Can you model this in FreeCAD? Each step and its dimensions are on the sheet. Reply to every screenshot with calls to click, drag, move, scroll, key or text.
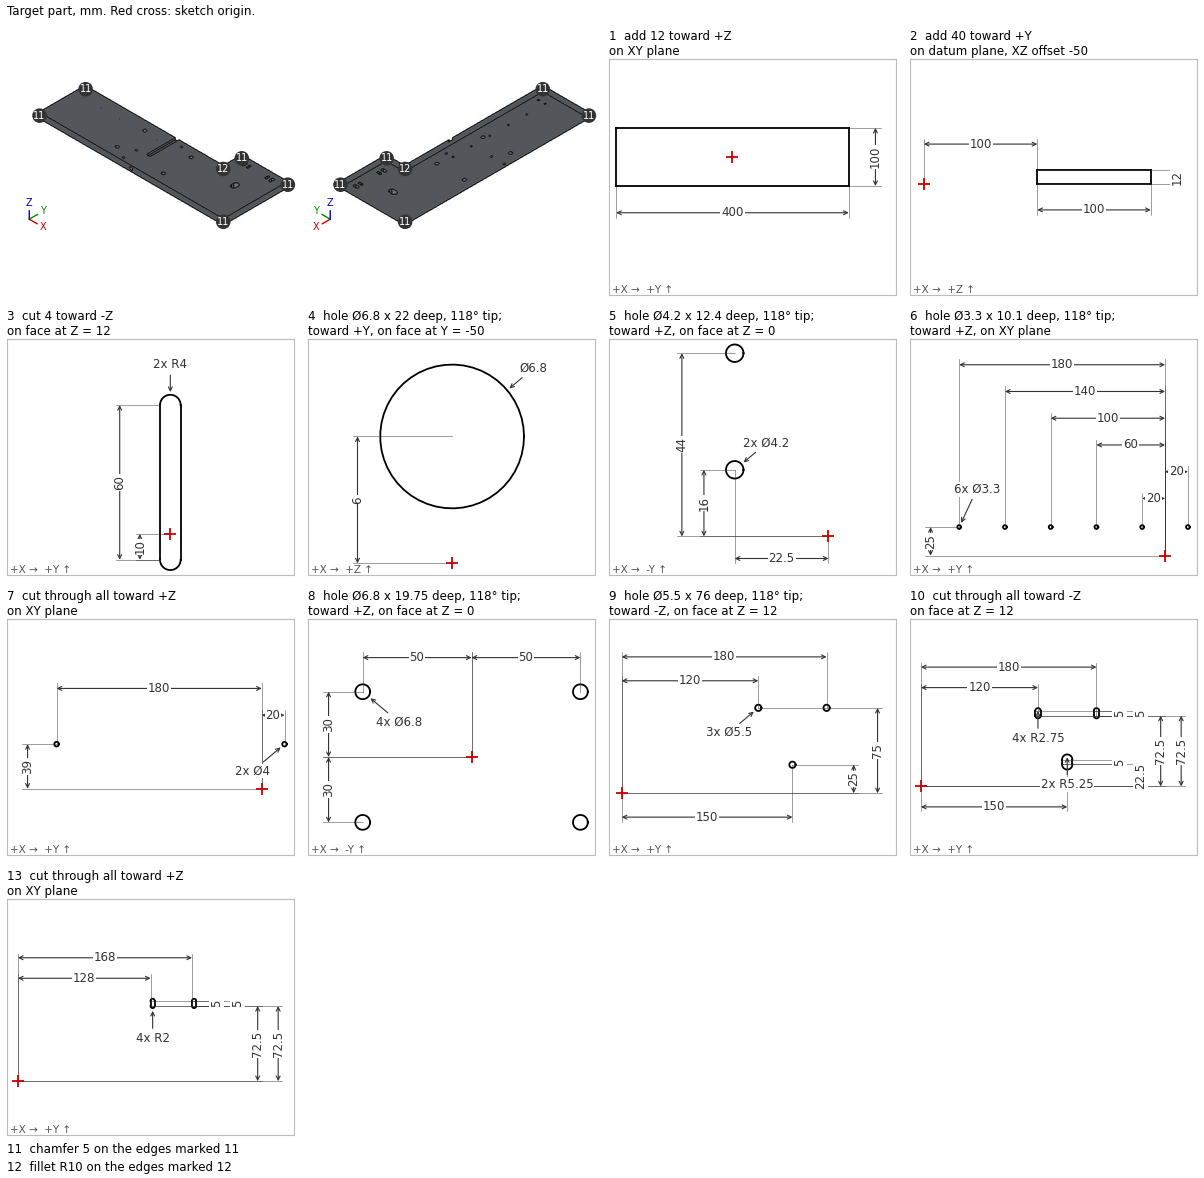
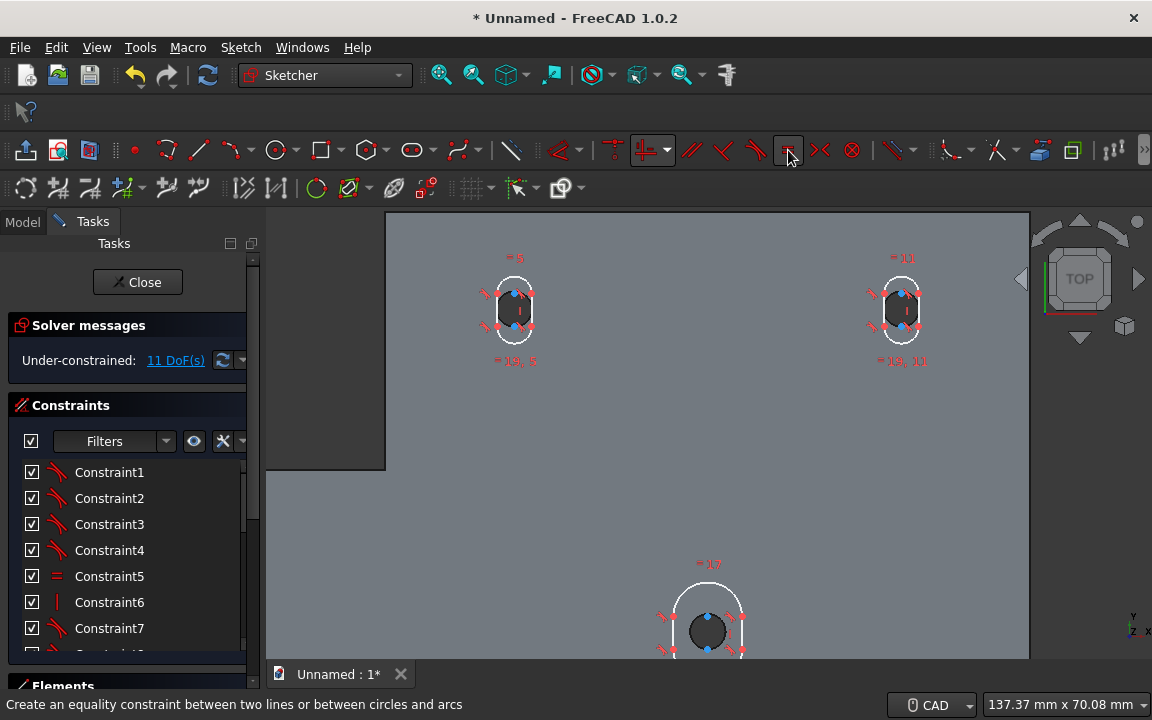
click(558, 150)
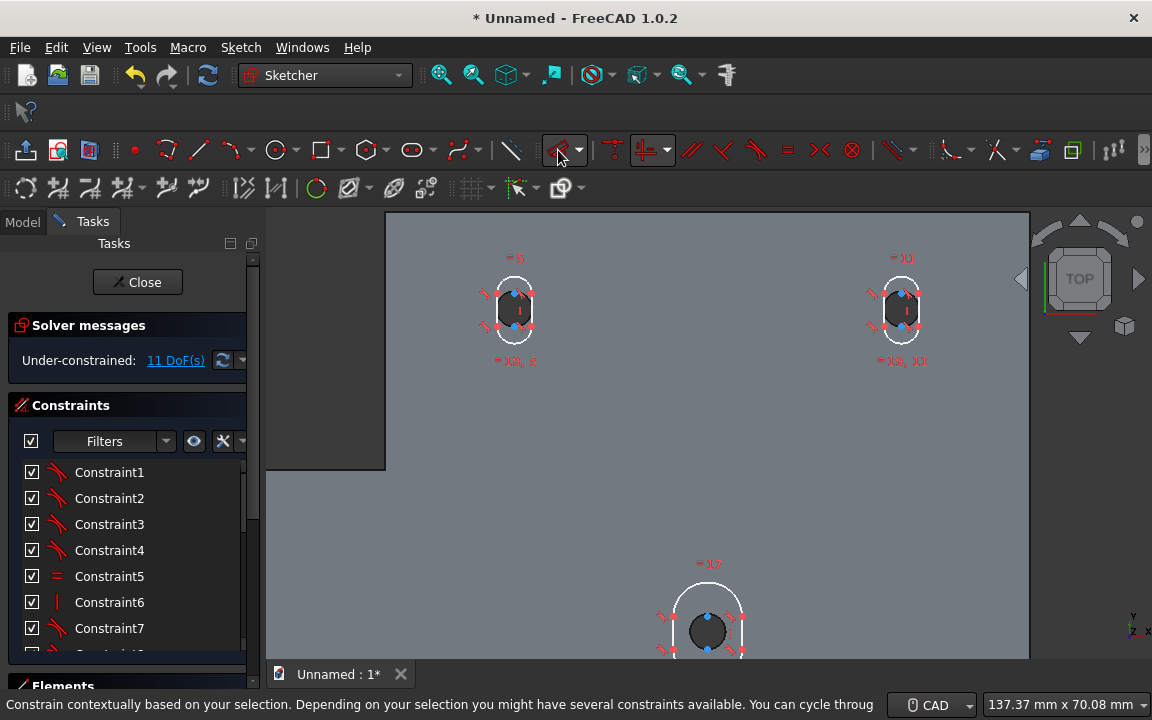
scroll(504, 340, up, 5)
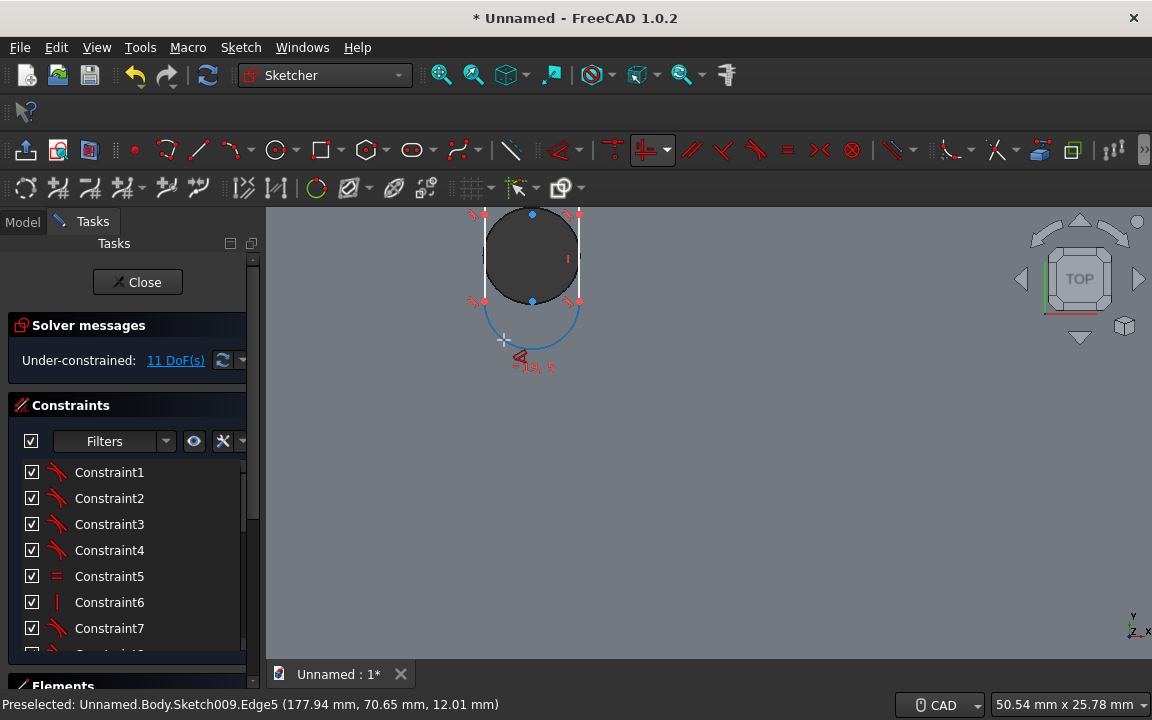
click(504, 340)
click(485, 366)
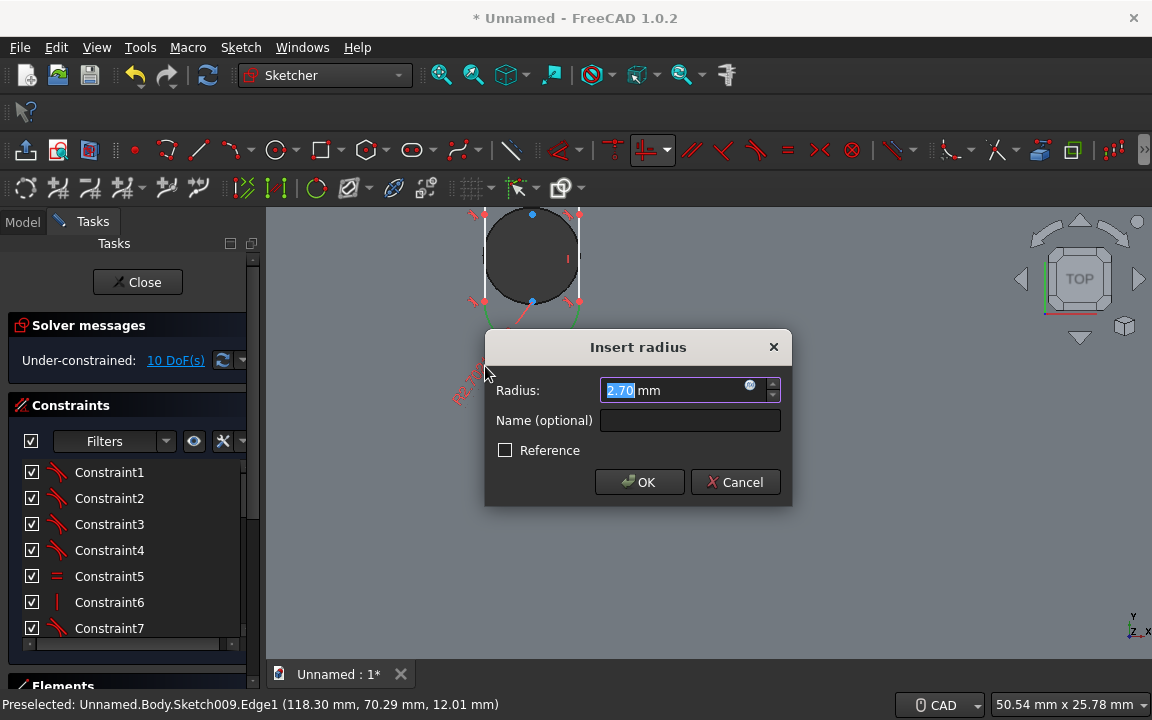
text(2.75)
key(Return)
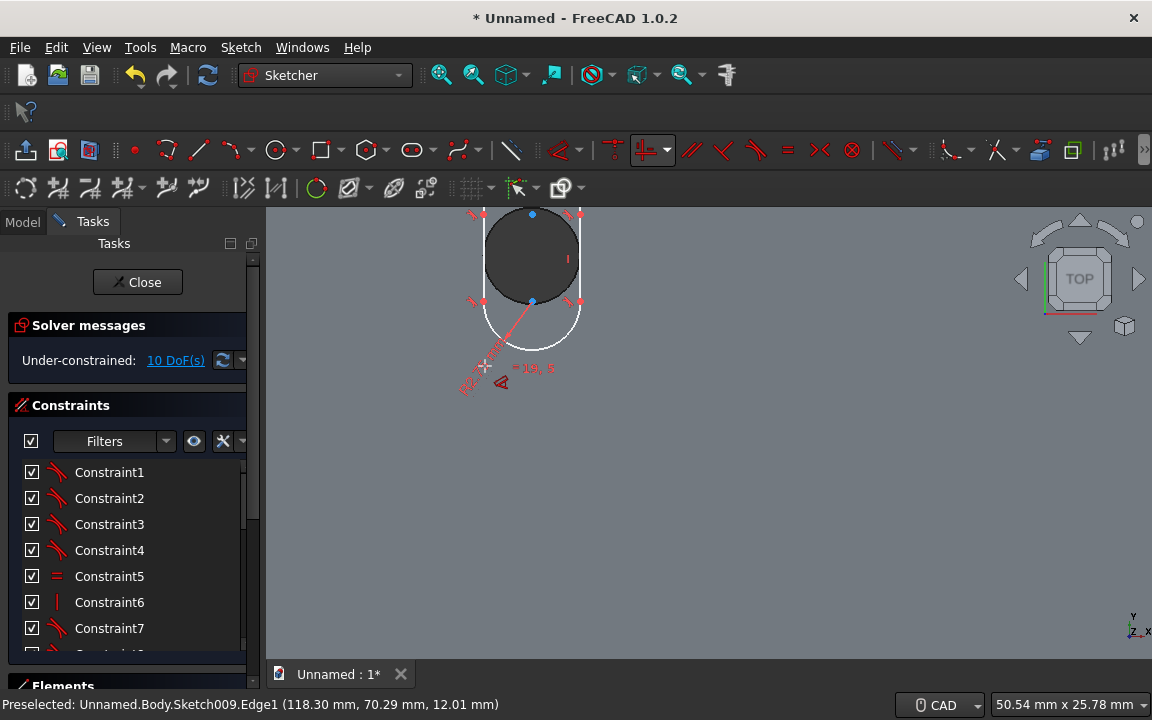
scroll(504, 340, down, 7)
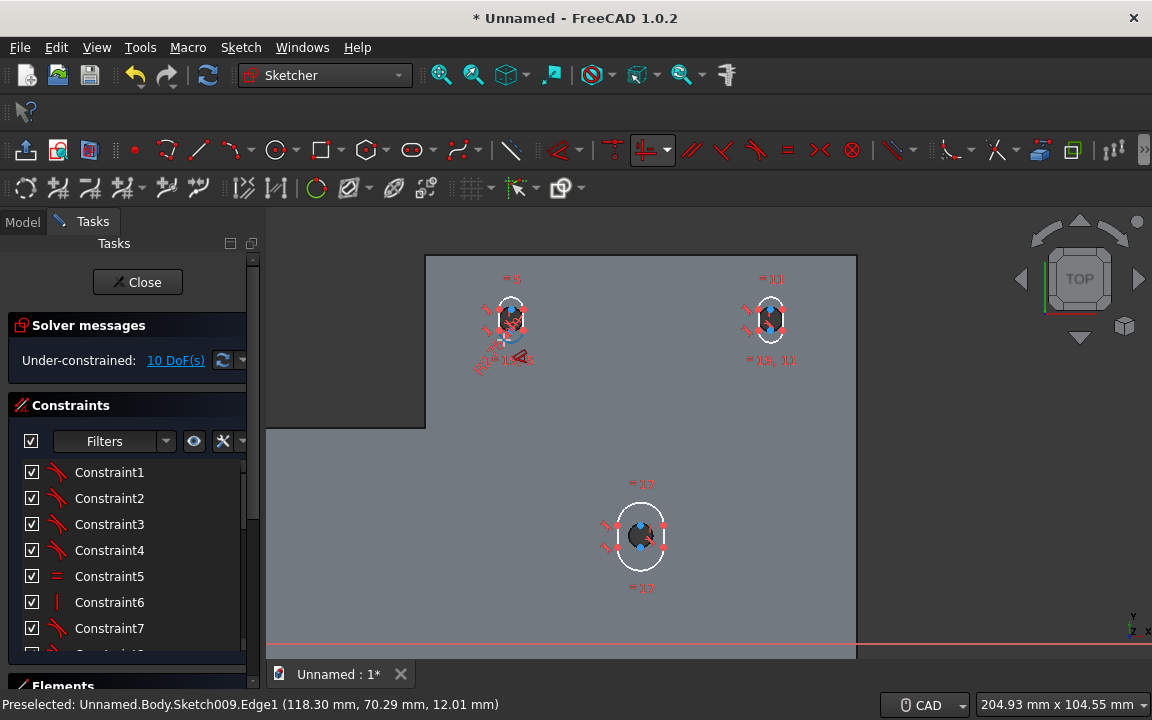
scroll(627, 566, up, 3)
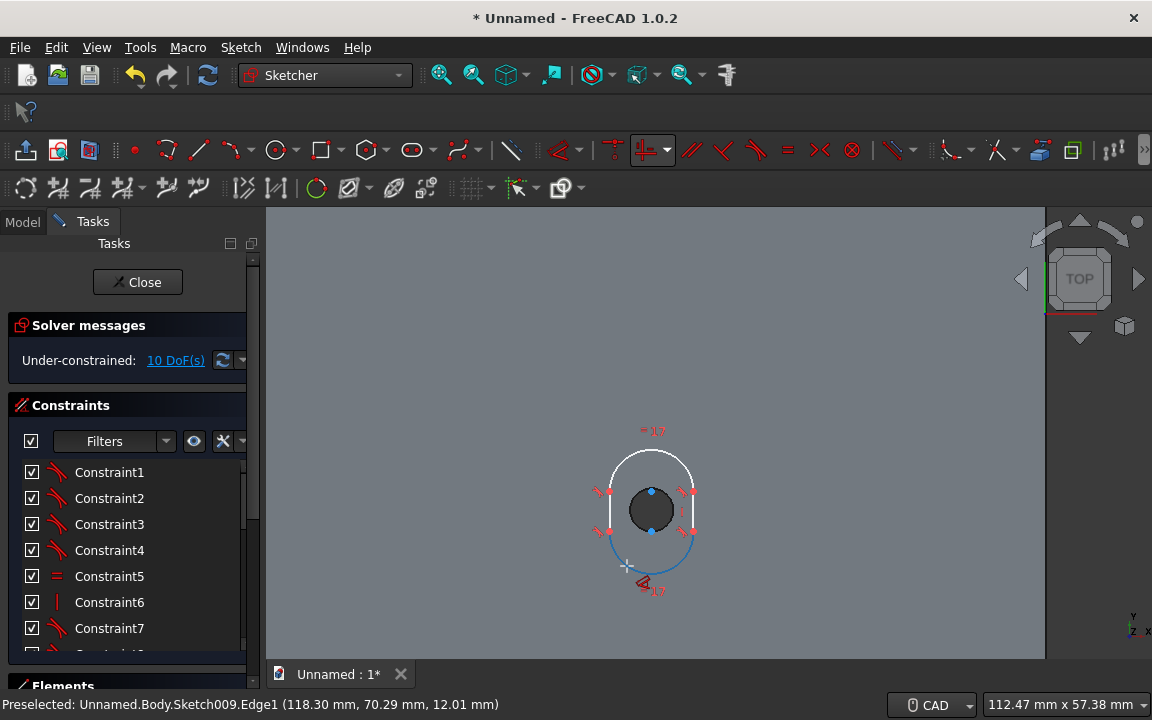
click(627, 566)
click(608, 592)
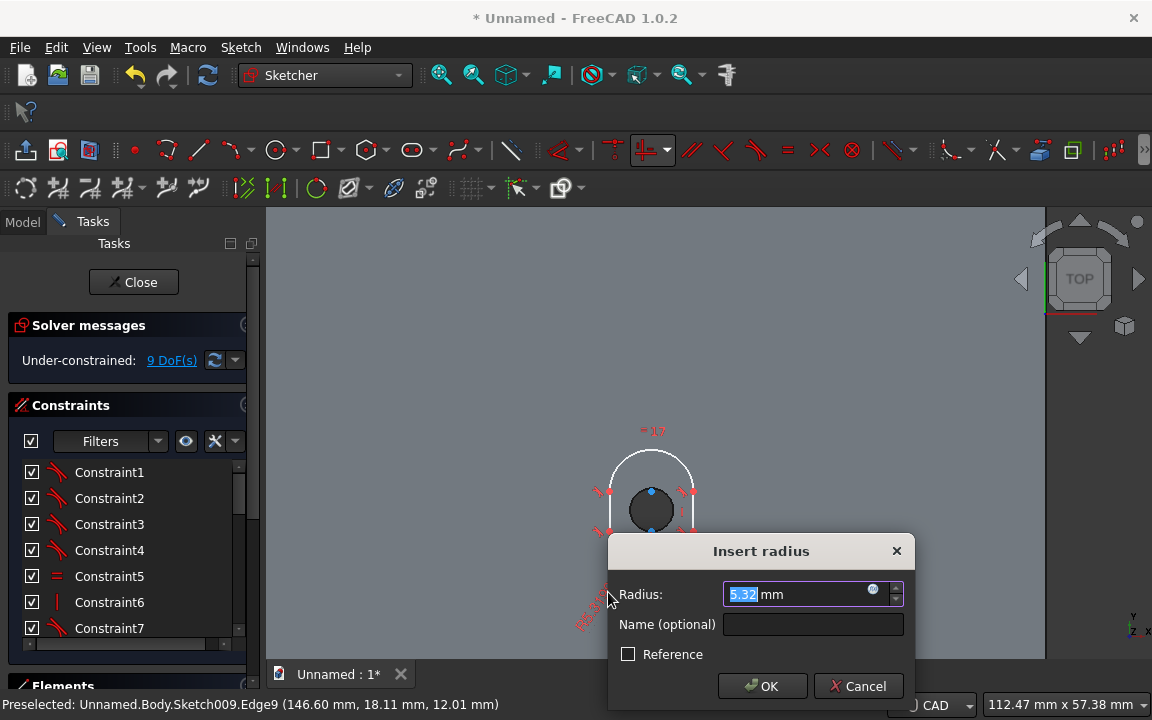
text(5.25)
key(Return)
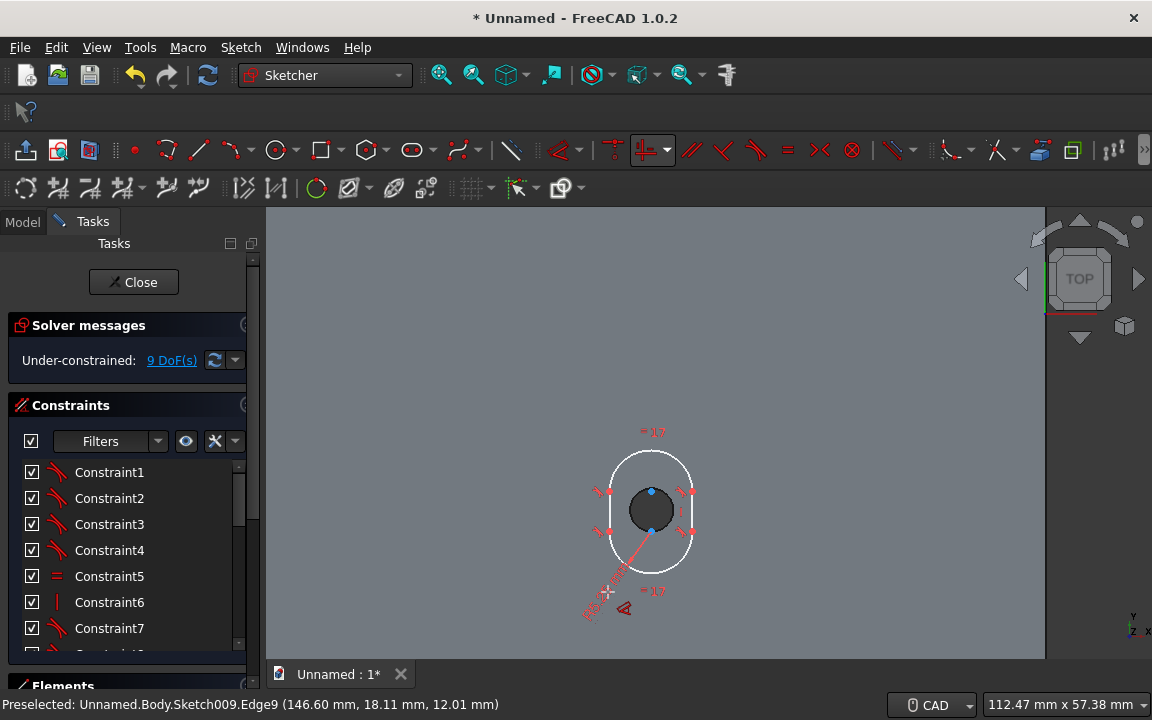
scroll(627, 567, down, 3)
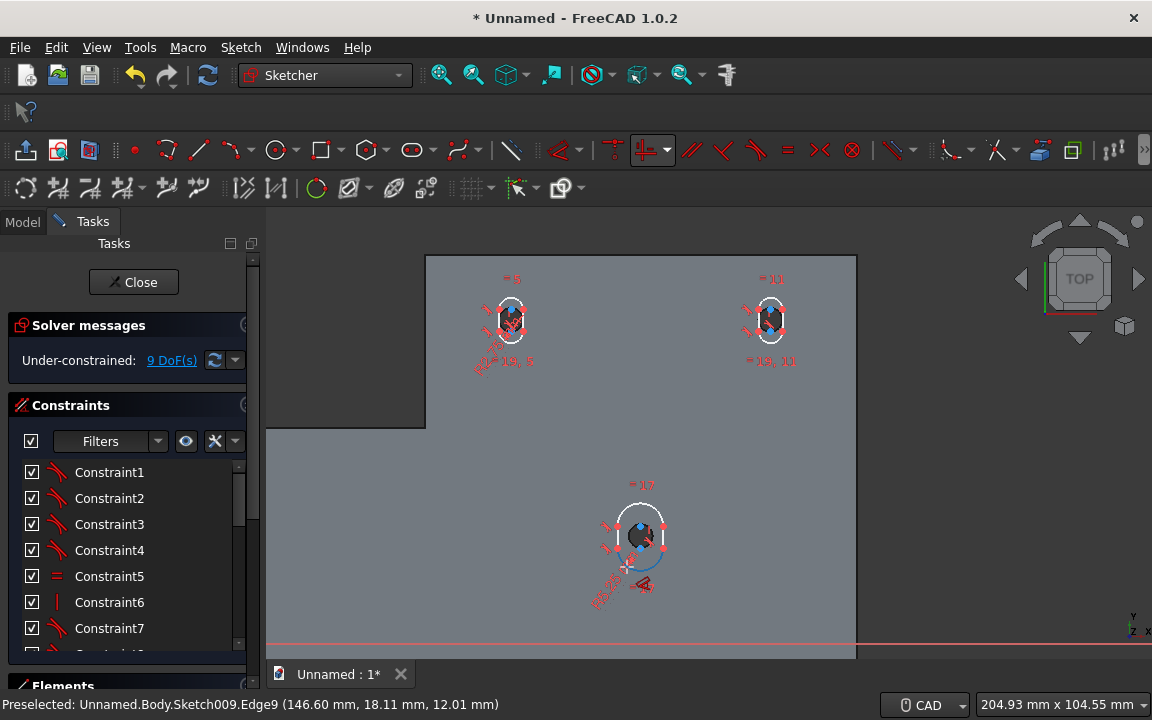
scroll(499, 325, up, 4)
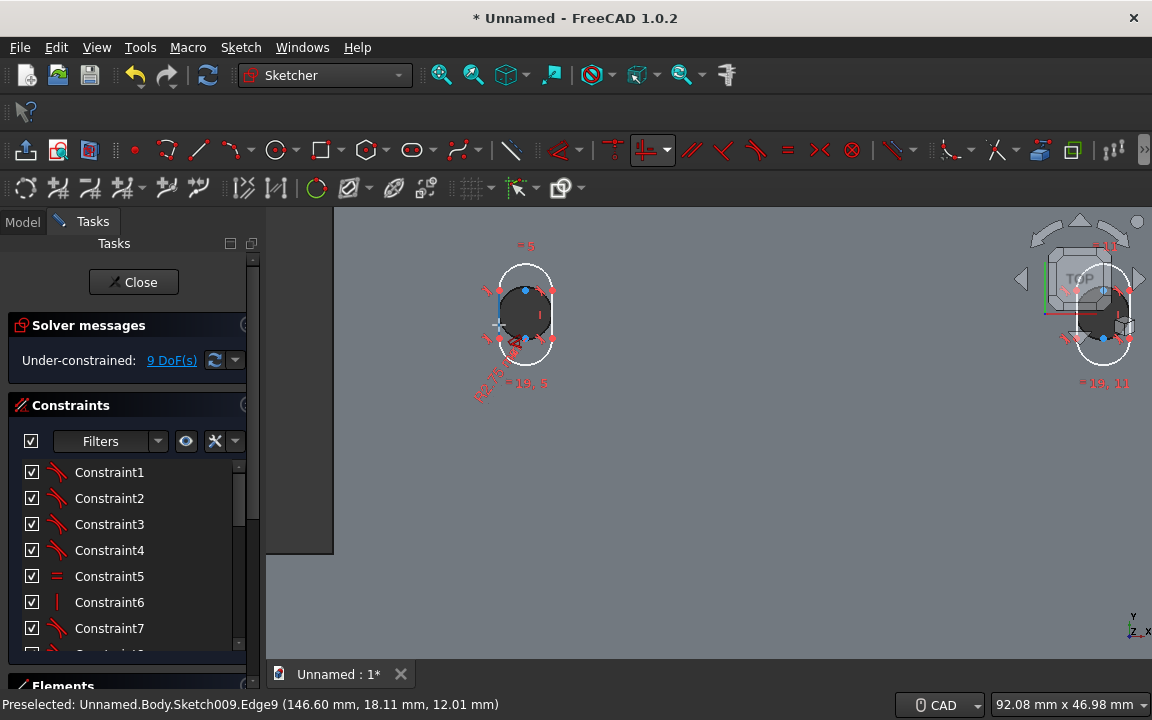
click(499, 324)
click(465, 315)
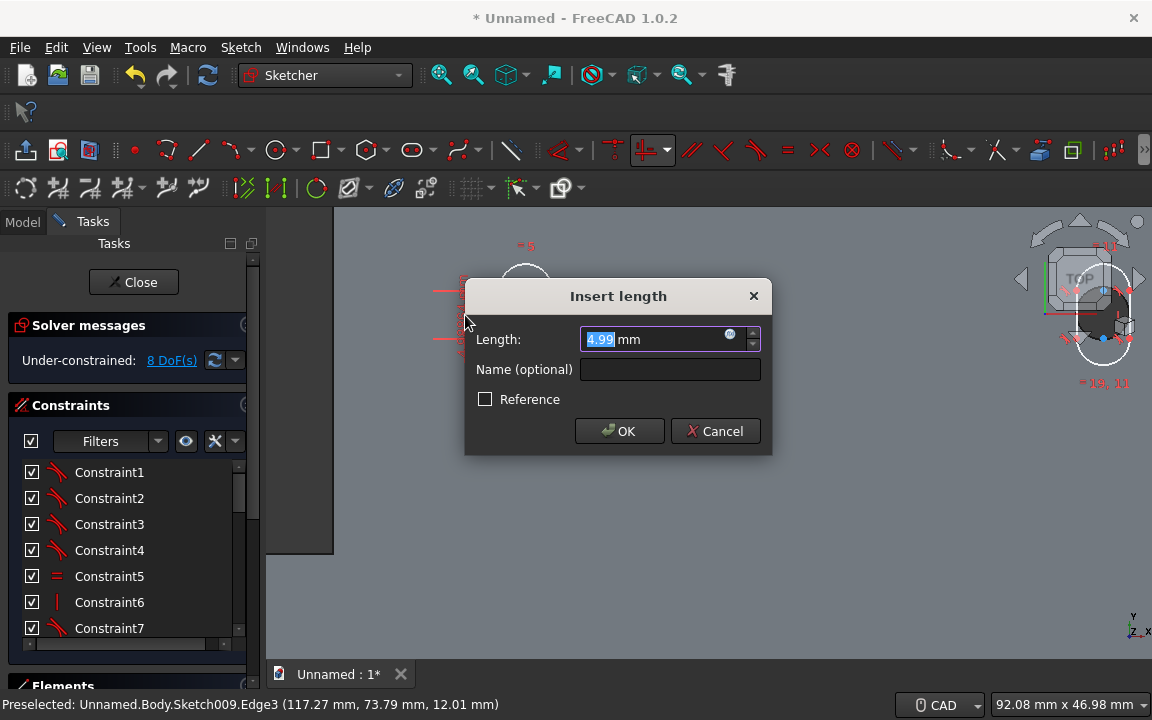
text(5)
key(Return)